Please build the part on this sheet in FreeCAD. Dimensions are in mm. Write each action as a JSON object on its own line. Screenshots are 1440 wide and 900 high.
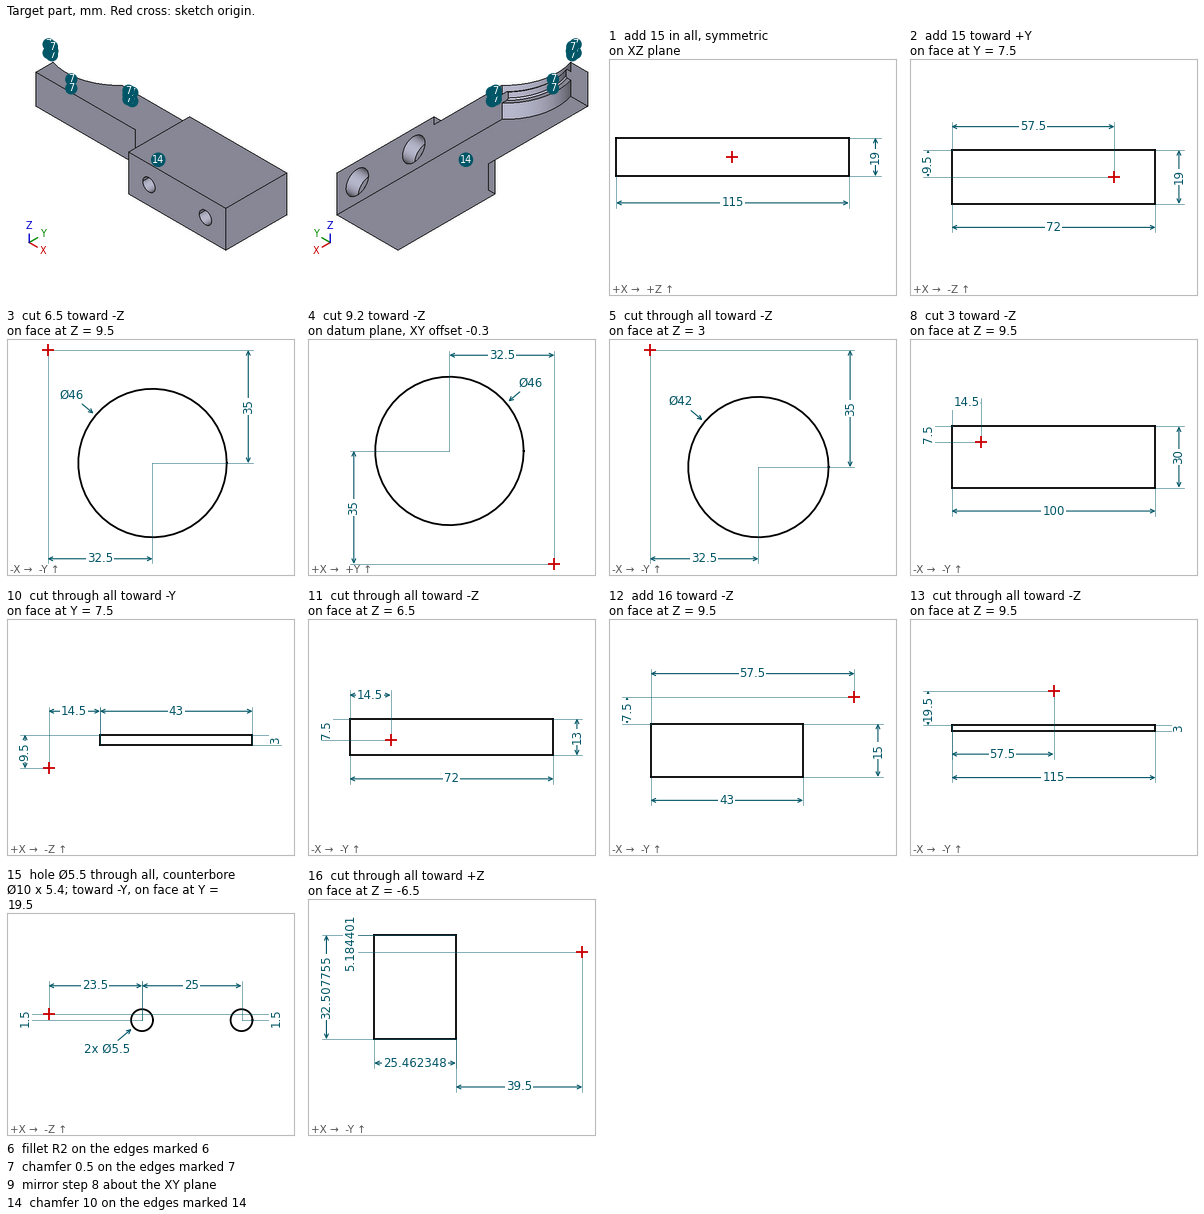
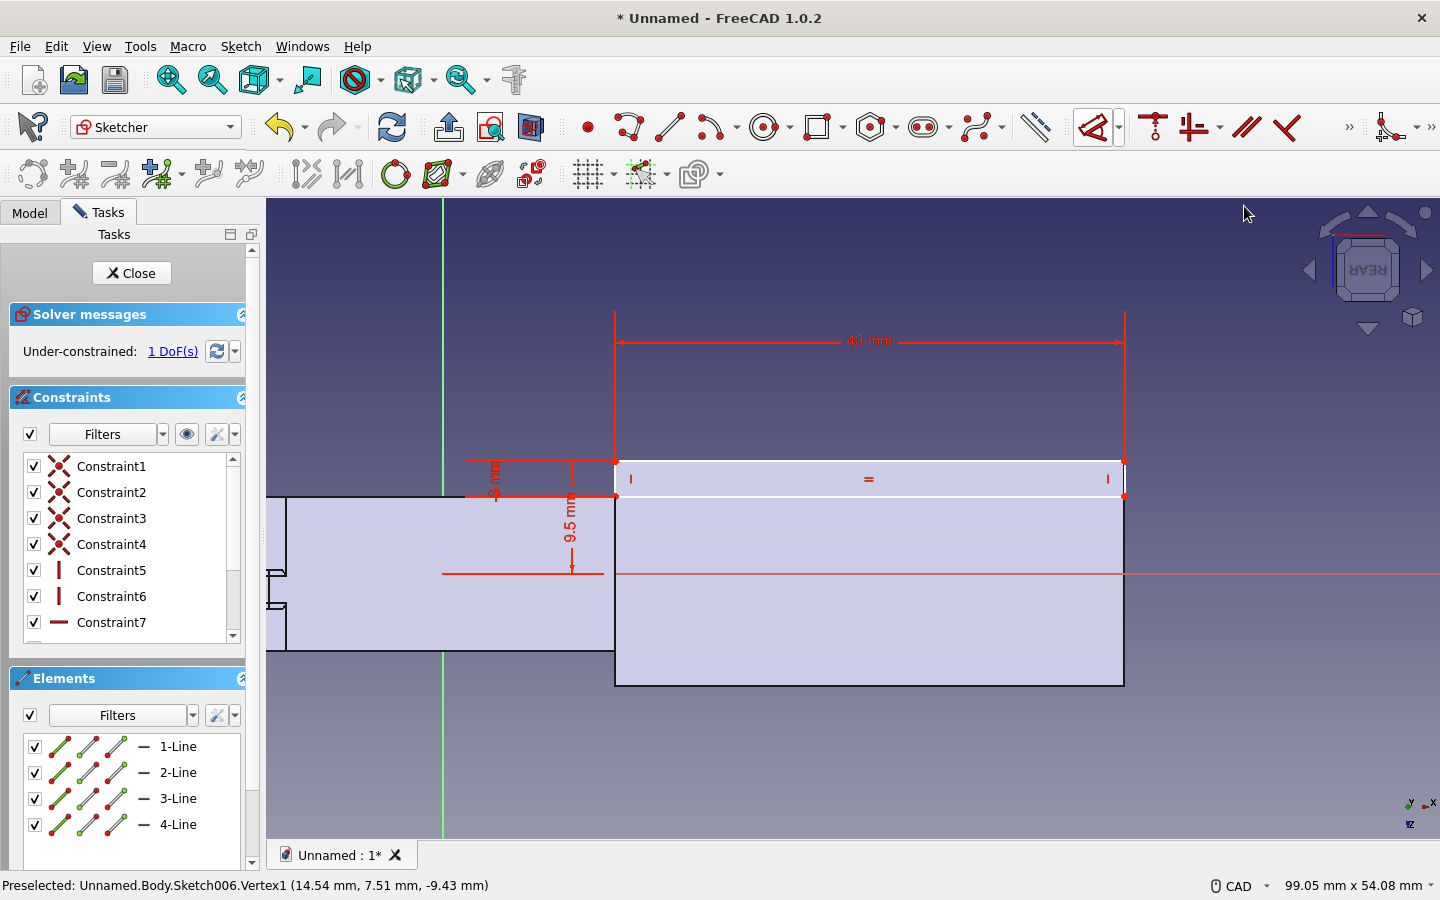
{"action": "left_click", "coordinate": [615, 461]}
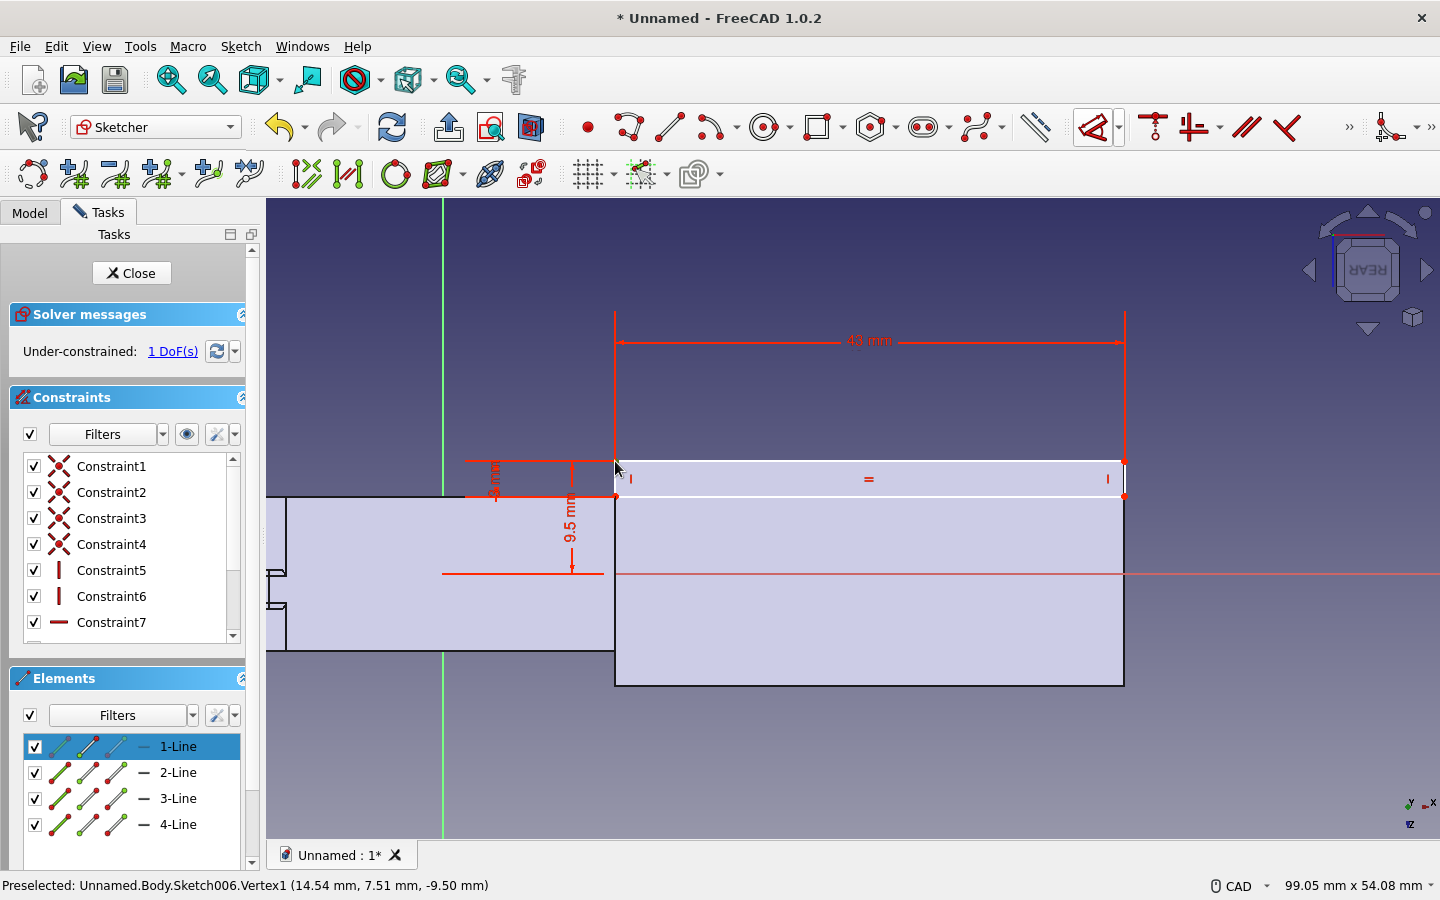
{"action": "left_click", "coordinate": [1118, 128]}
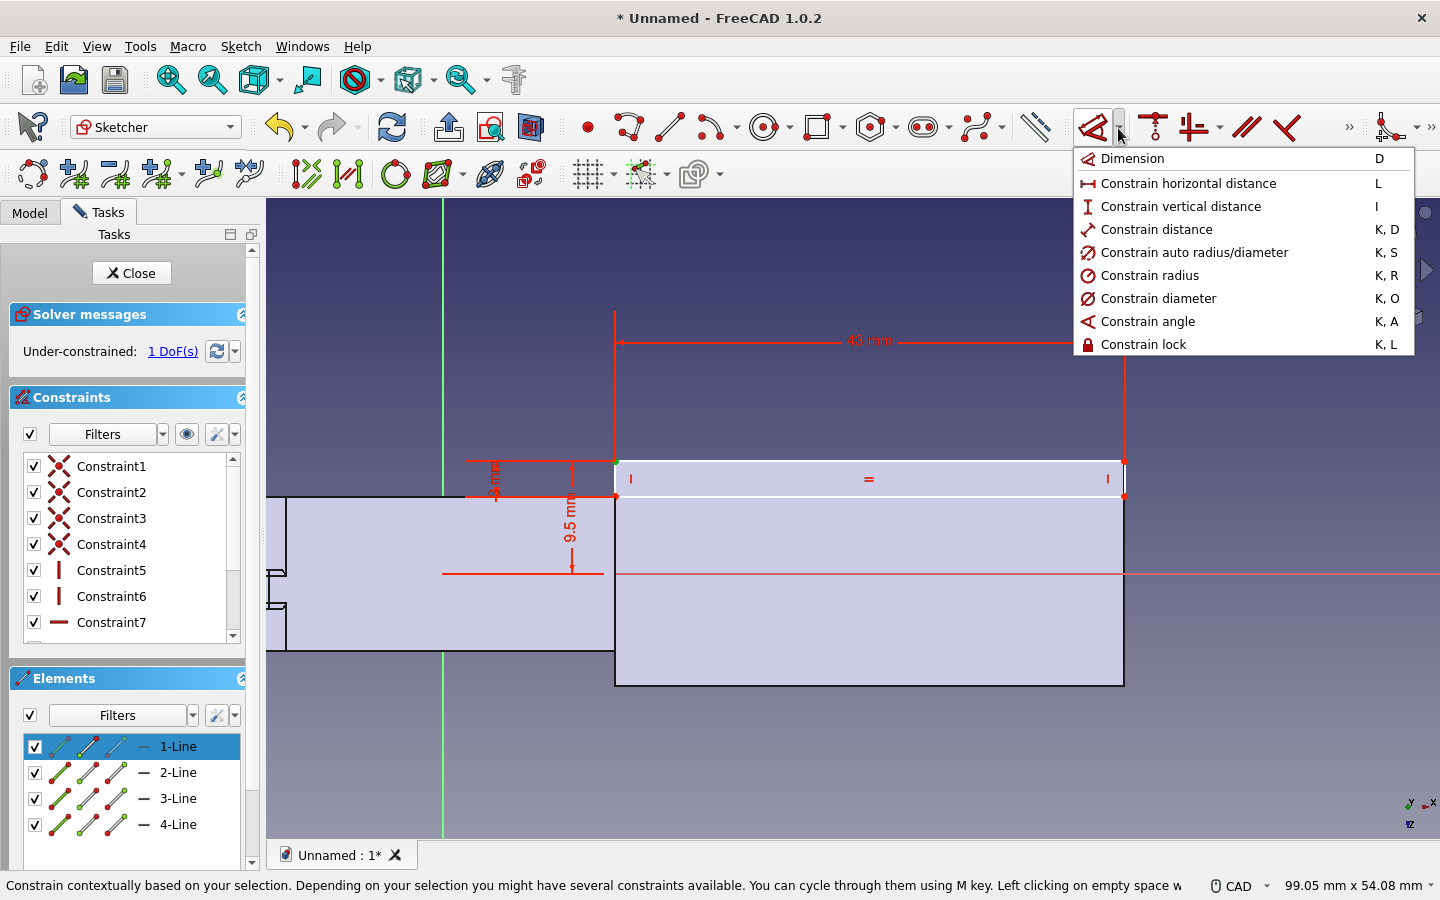
{"action": "left_click", "coordinate": [1244, 184]}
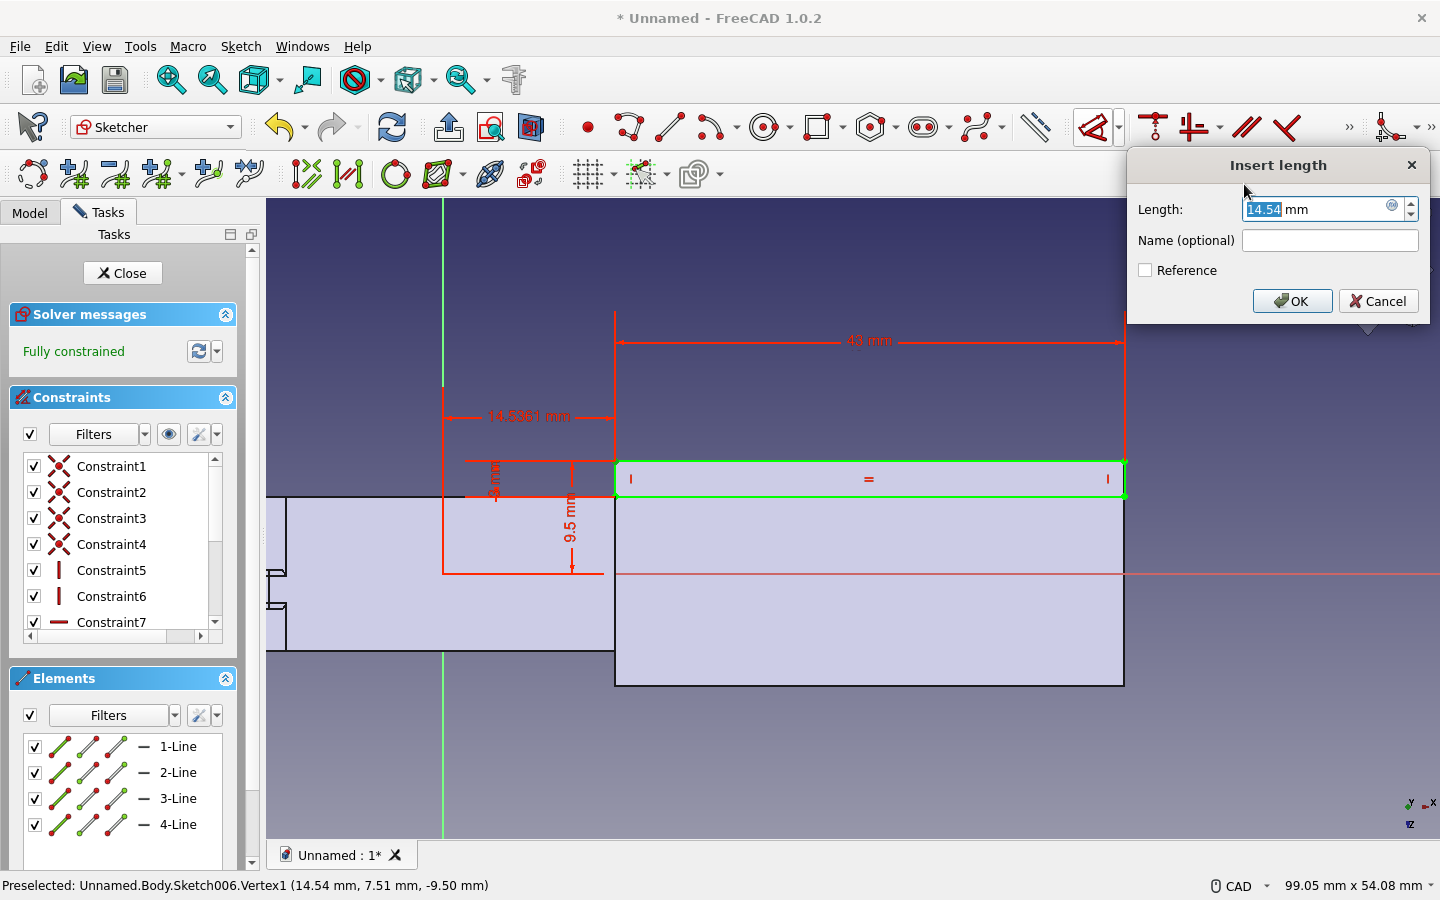
{"action": "type", "text": "14.5"}
{"action": "key", "text": "Return"}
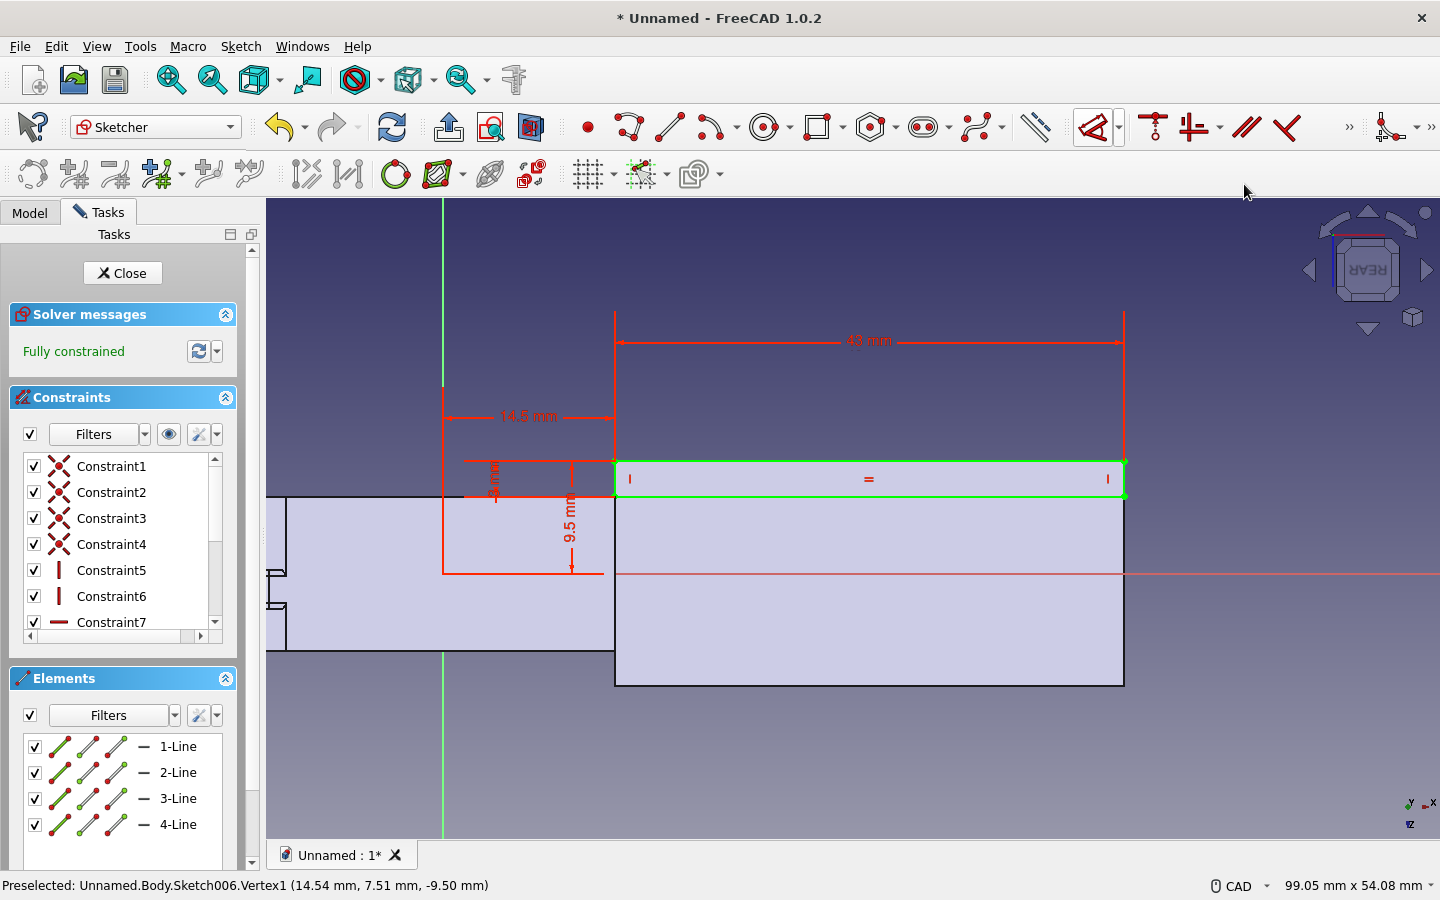
{"action": "left_click", "coordinate": [123, 273]}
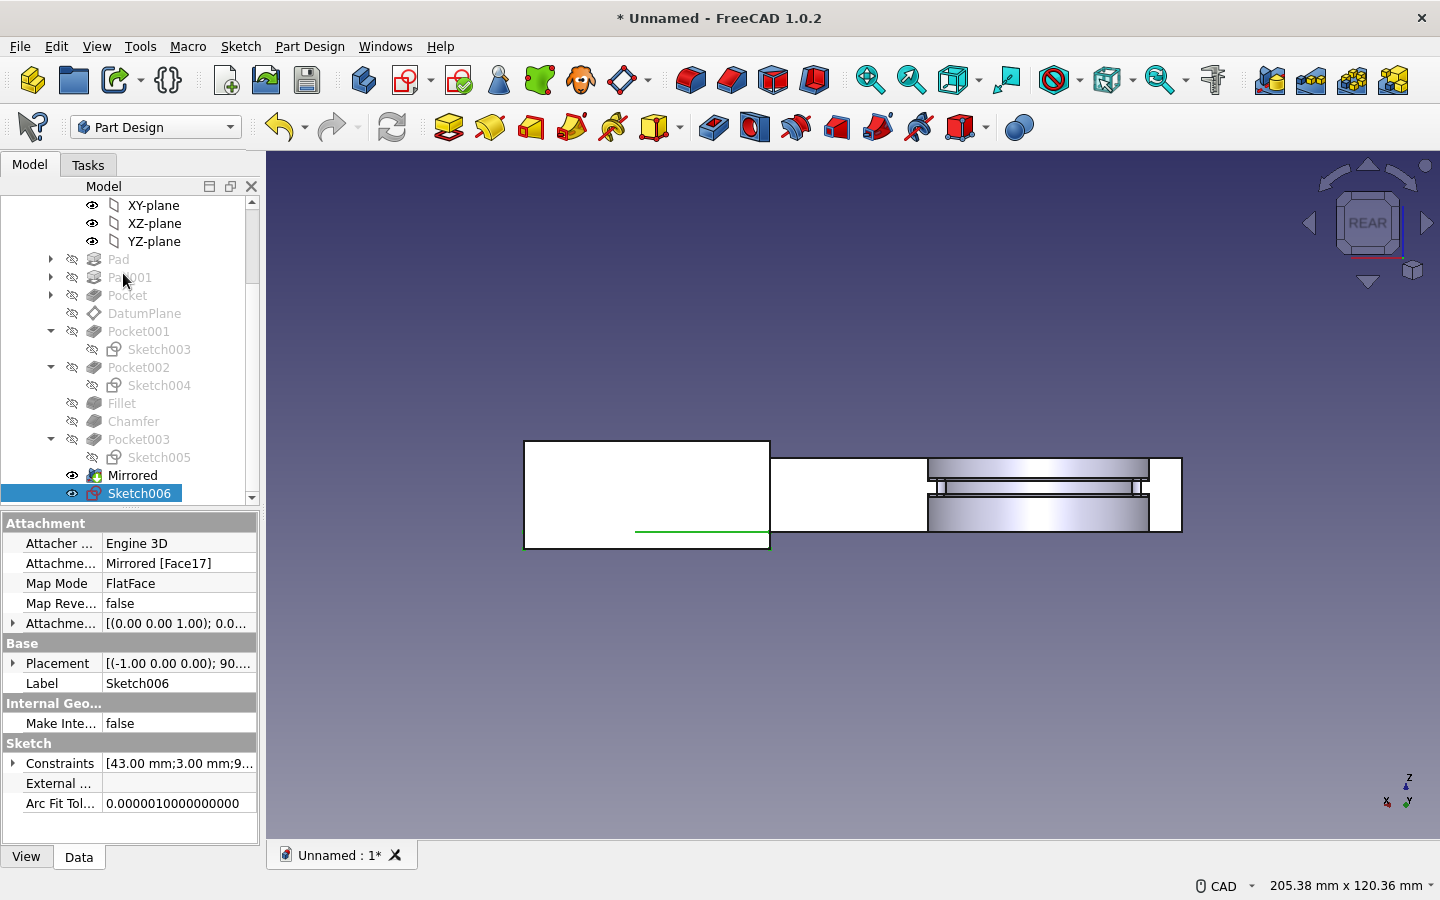
{"action": "left_click", "coordinate": [714, 128]}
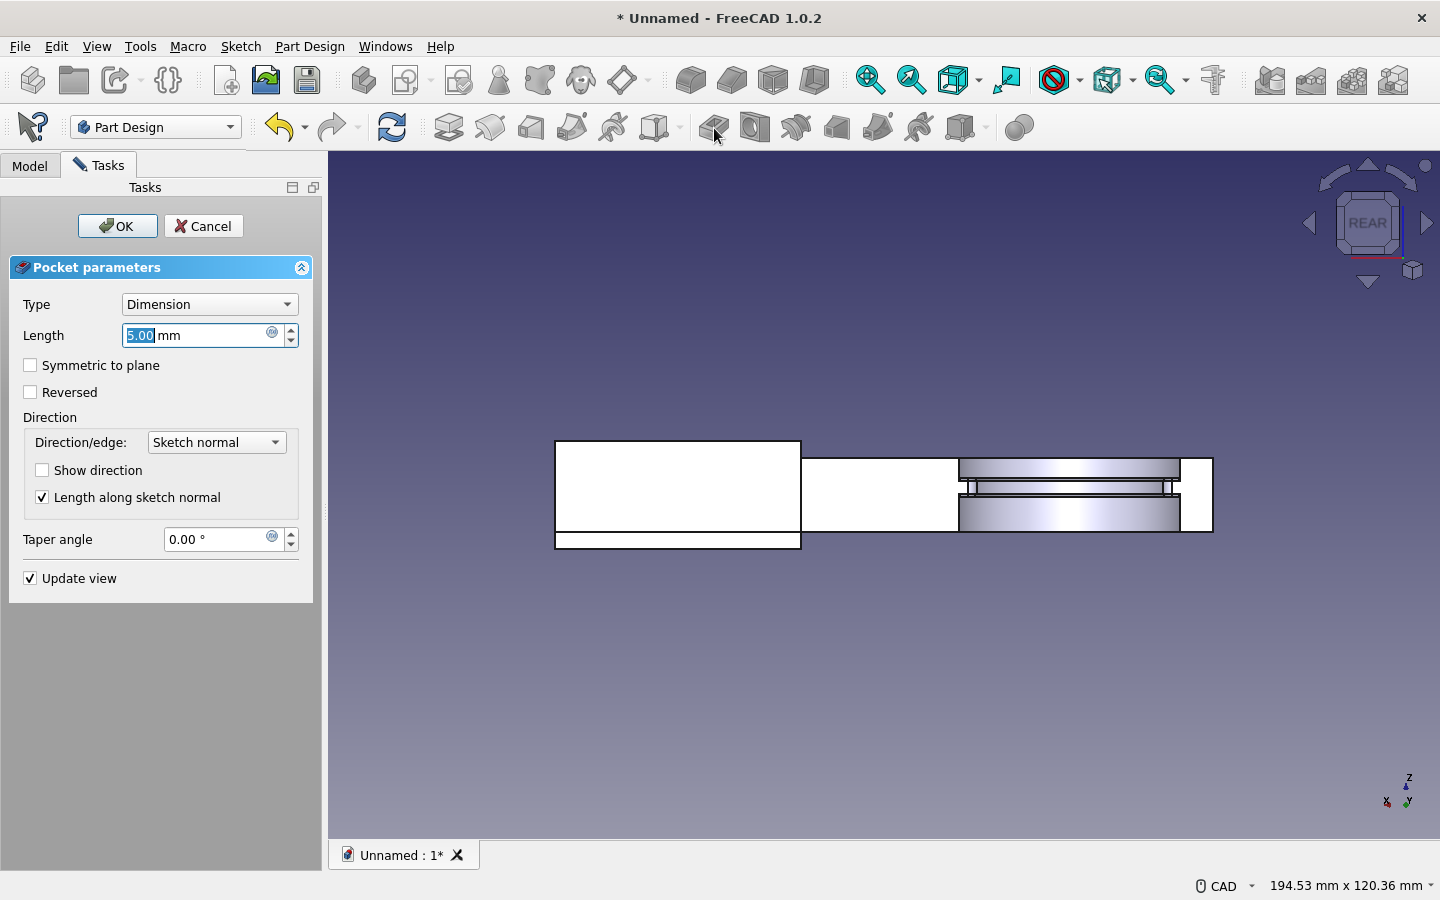
{"action": "left_click", "coordinate": [210, 304]}